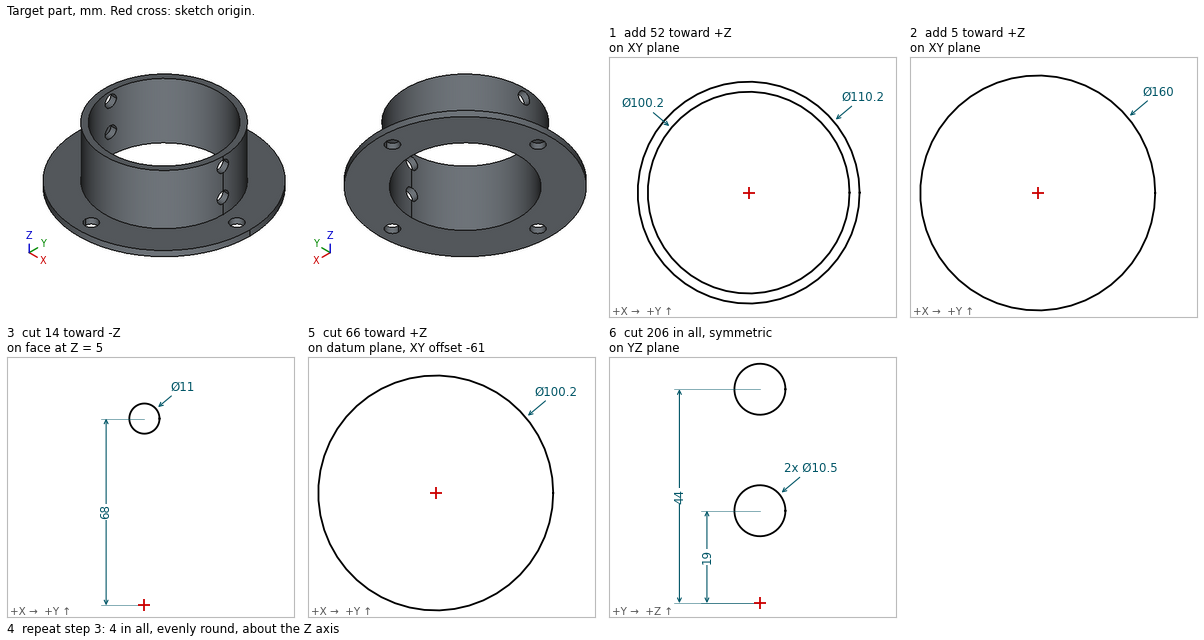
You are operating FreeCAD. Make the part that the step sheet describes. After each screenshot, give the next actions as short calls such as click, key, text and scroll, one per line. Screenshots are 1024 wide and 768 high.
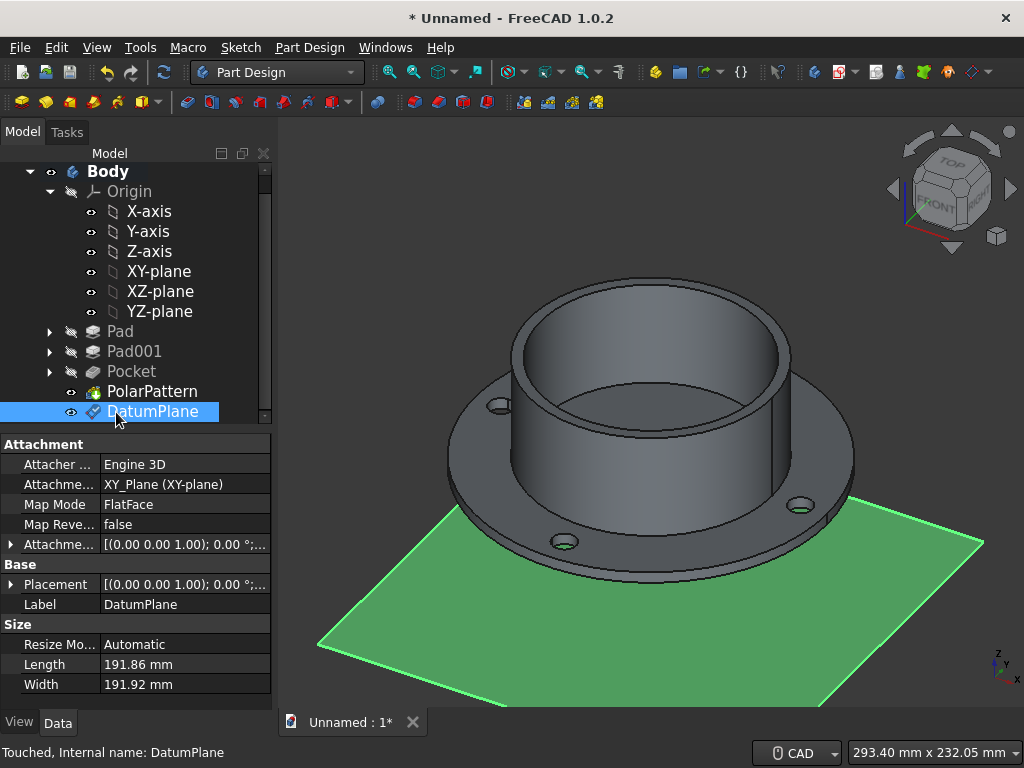
click(840, 72)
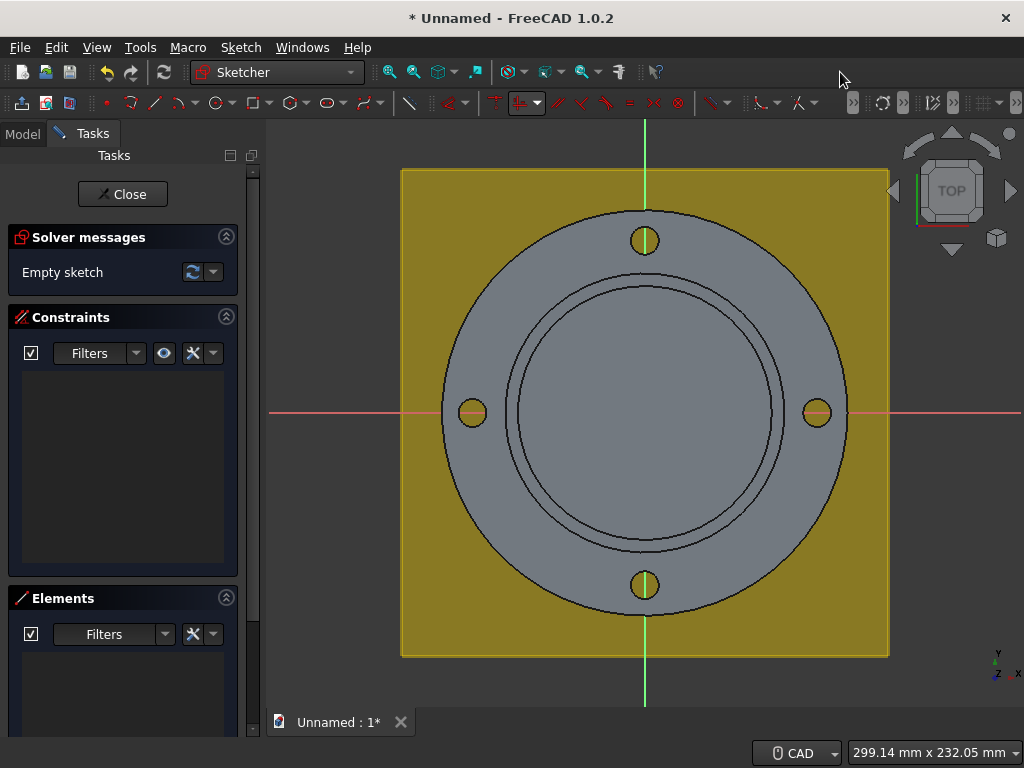
click(70, 104)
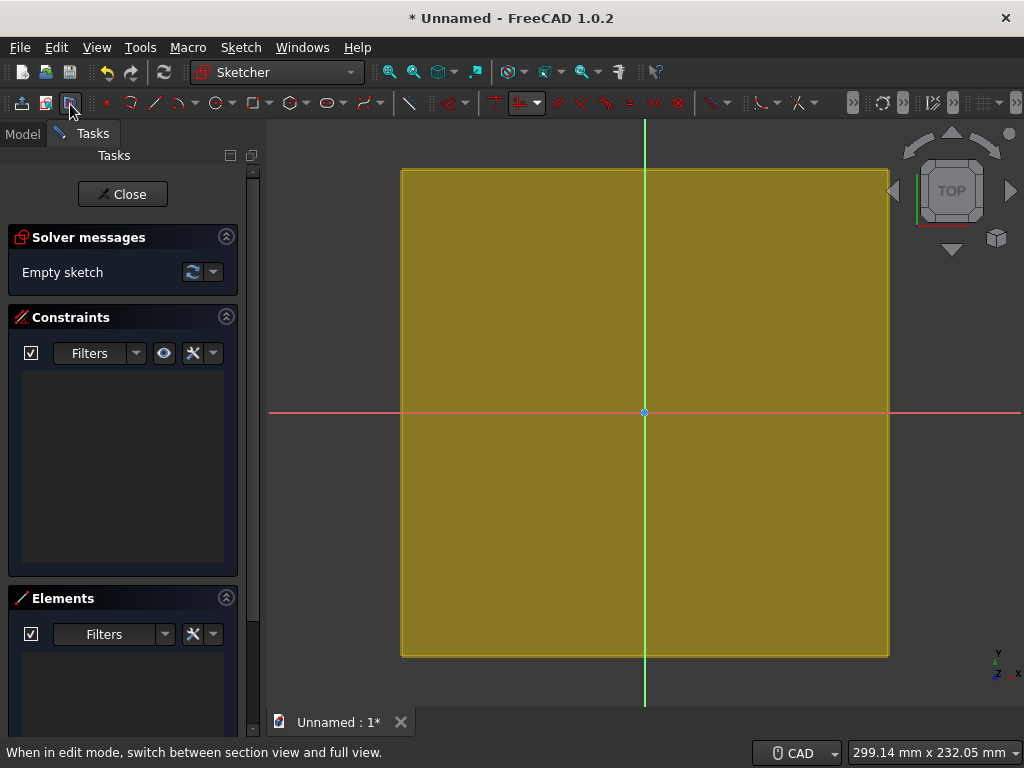
scroll(784, 413, up, 2)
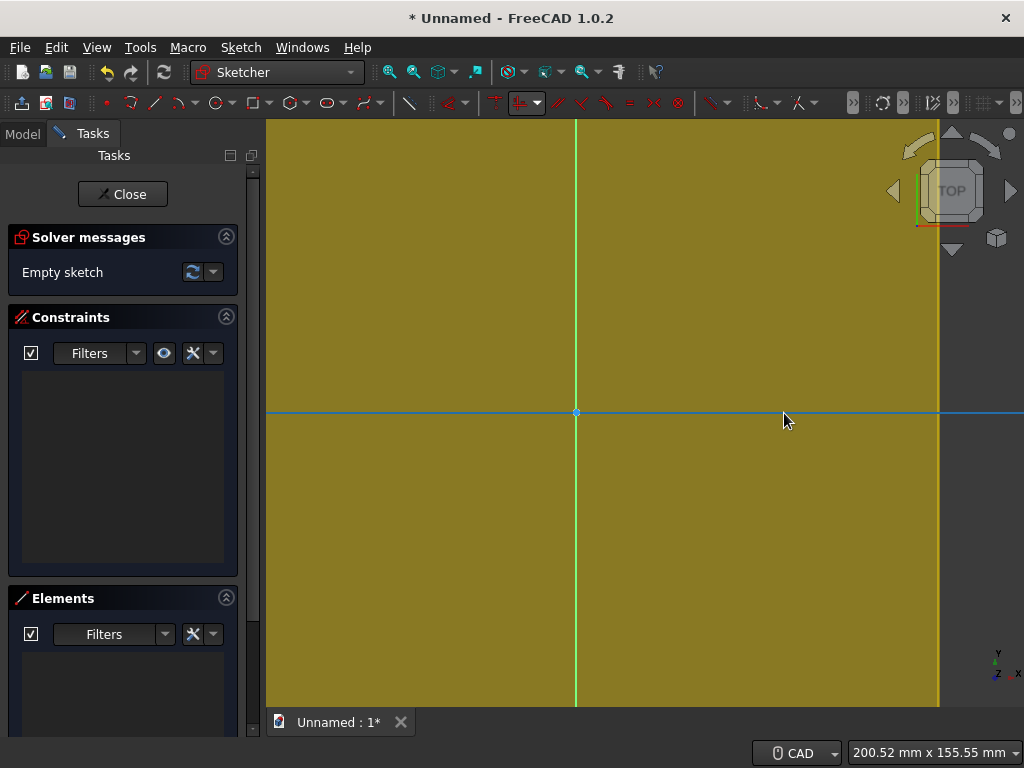
click(216, 104)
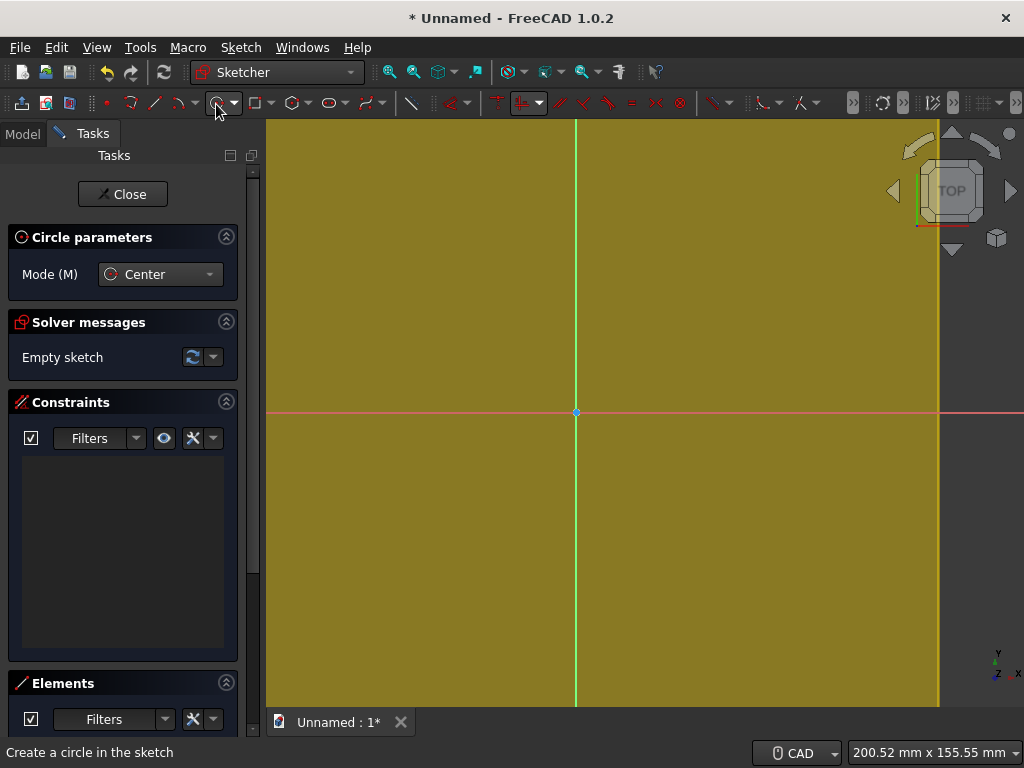
click(576, 413)
click(710, 279)
key(Escape)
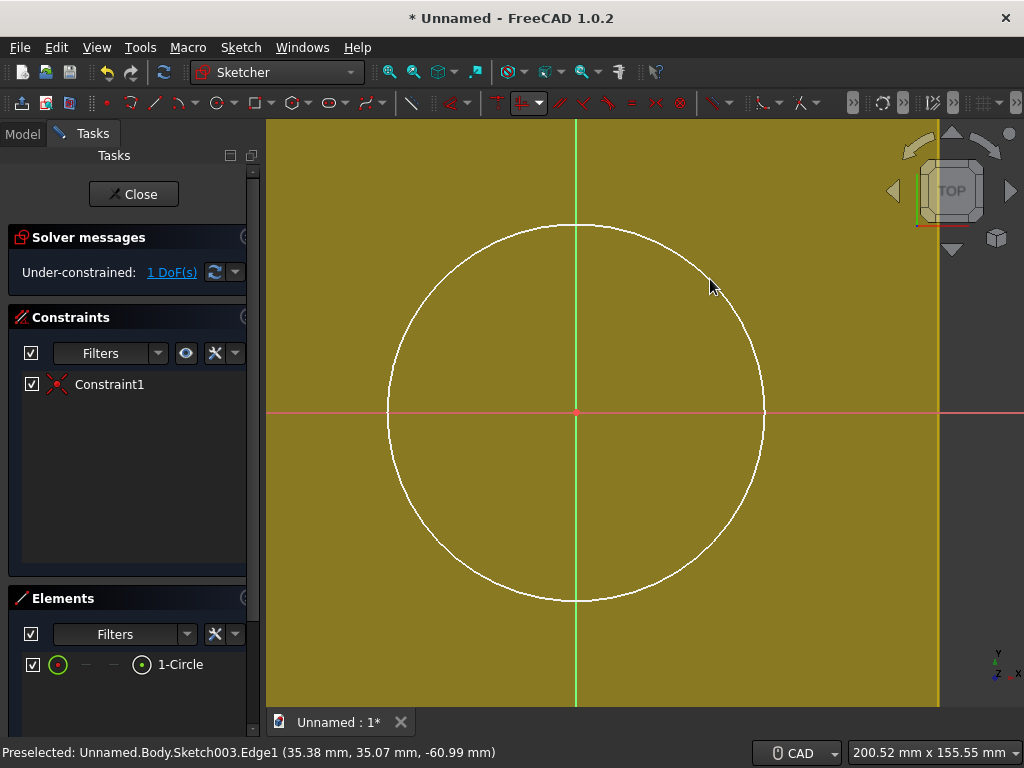
click(450, 104)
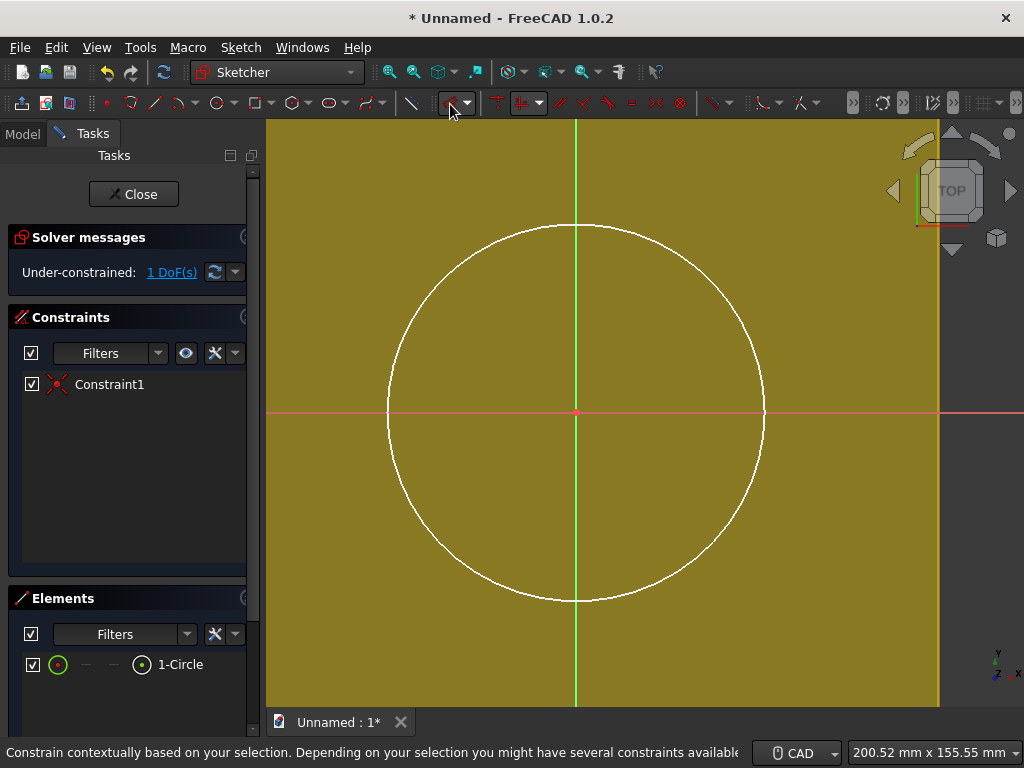
click(709, 279)
click(732, 256)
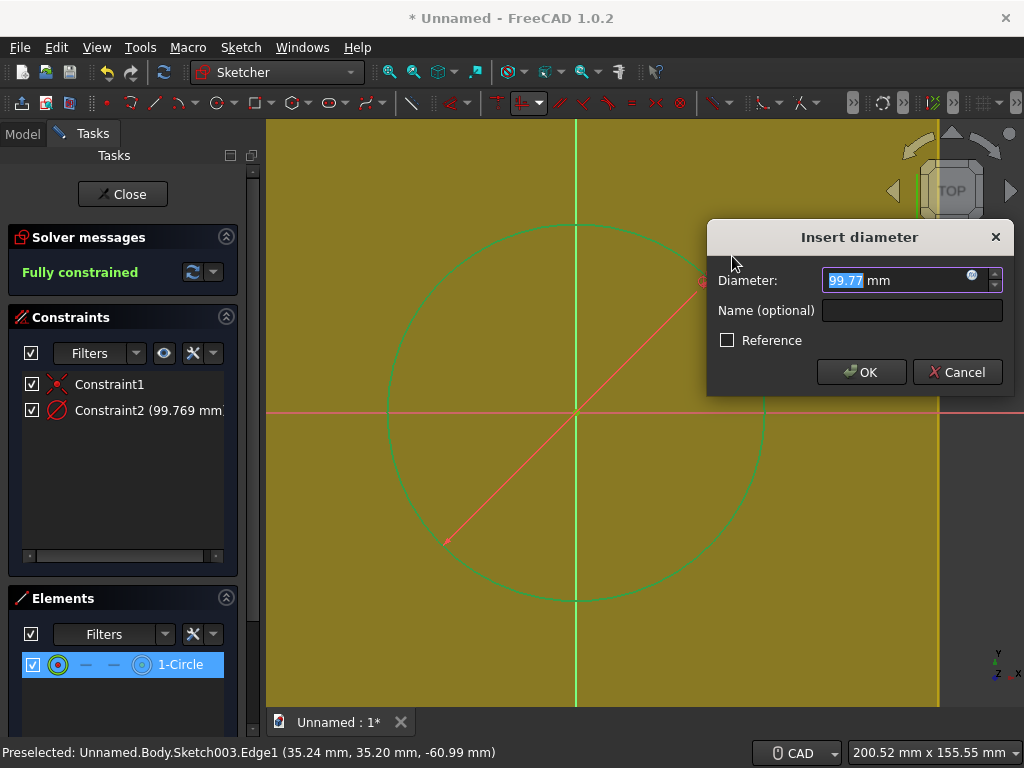
text(100.2)
key(Return)
key(Escape)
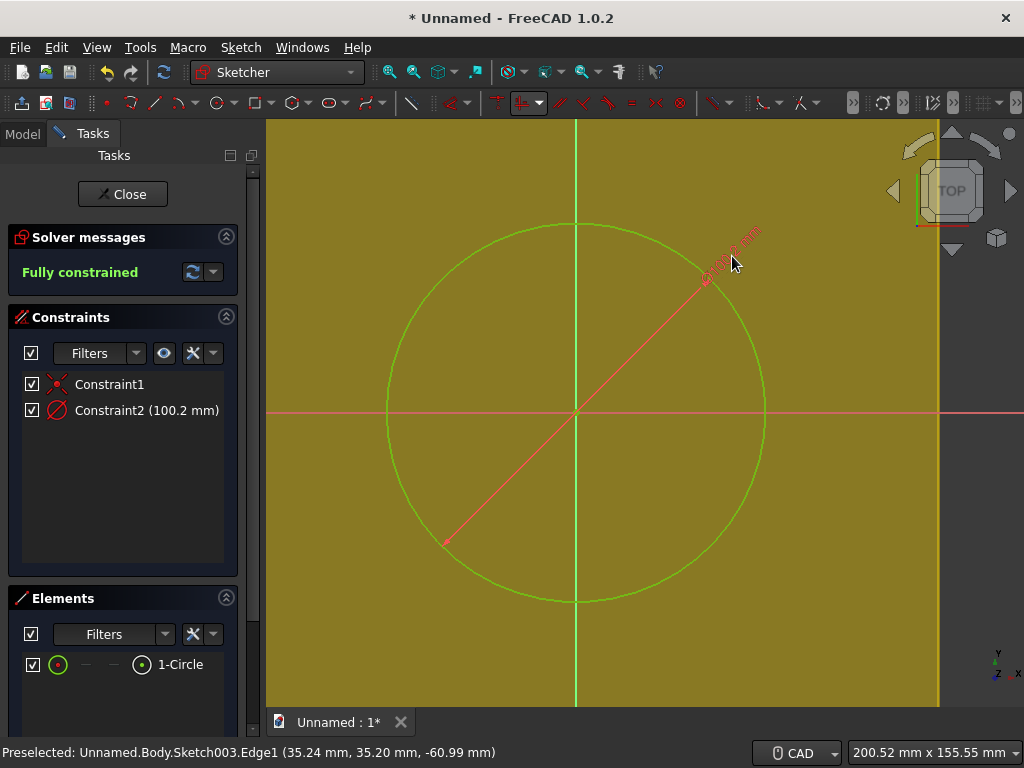
click(123, 194)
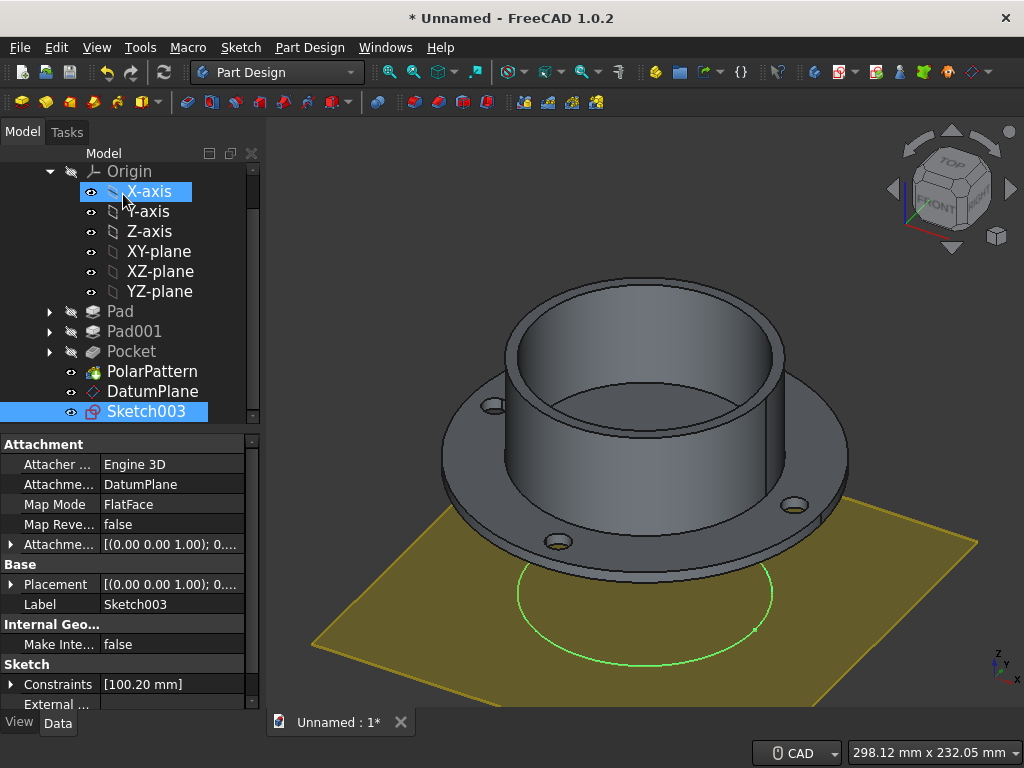
click(188, 102)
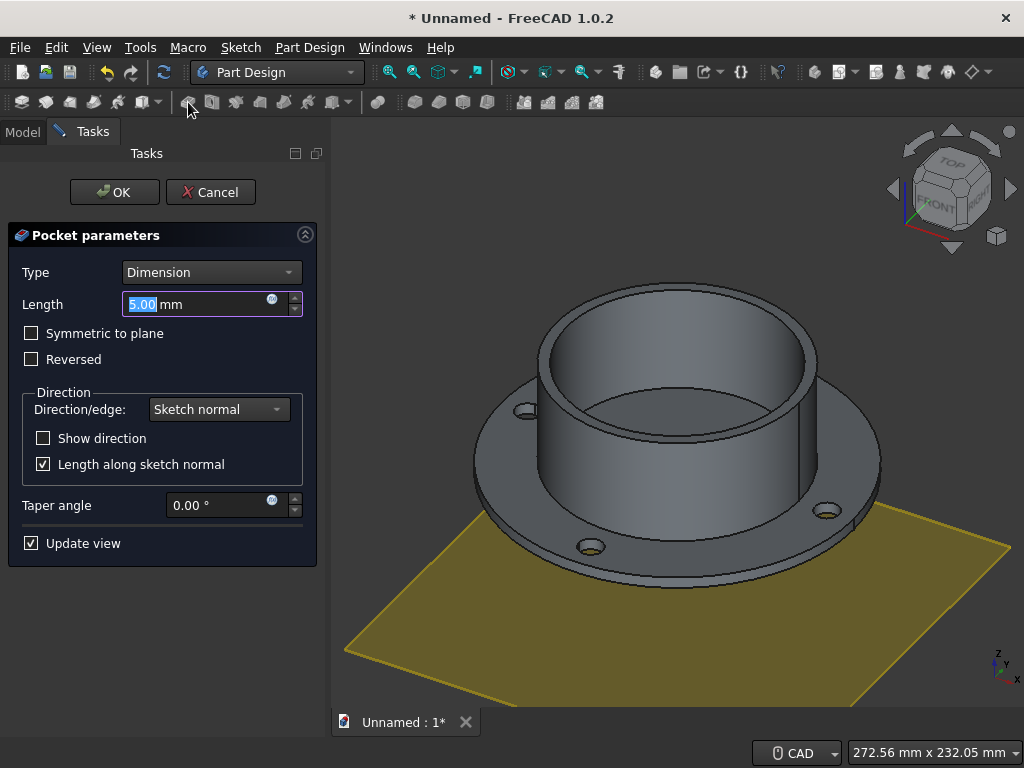
text(66)
key(Tab)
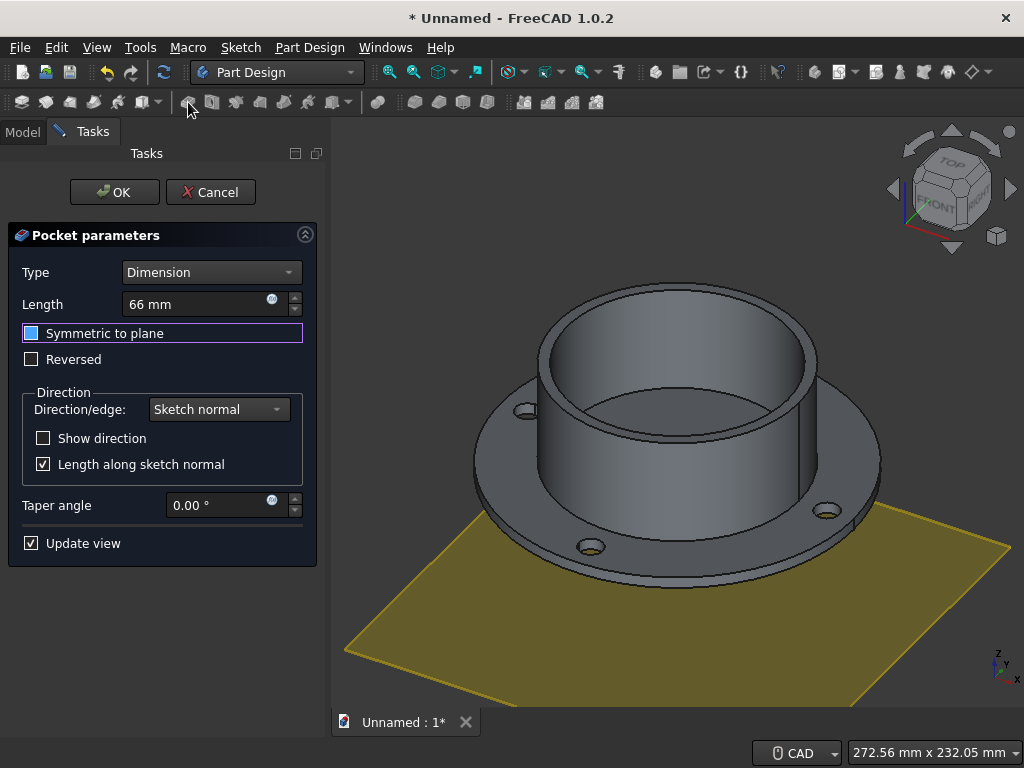
click(30, 359)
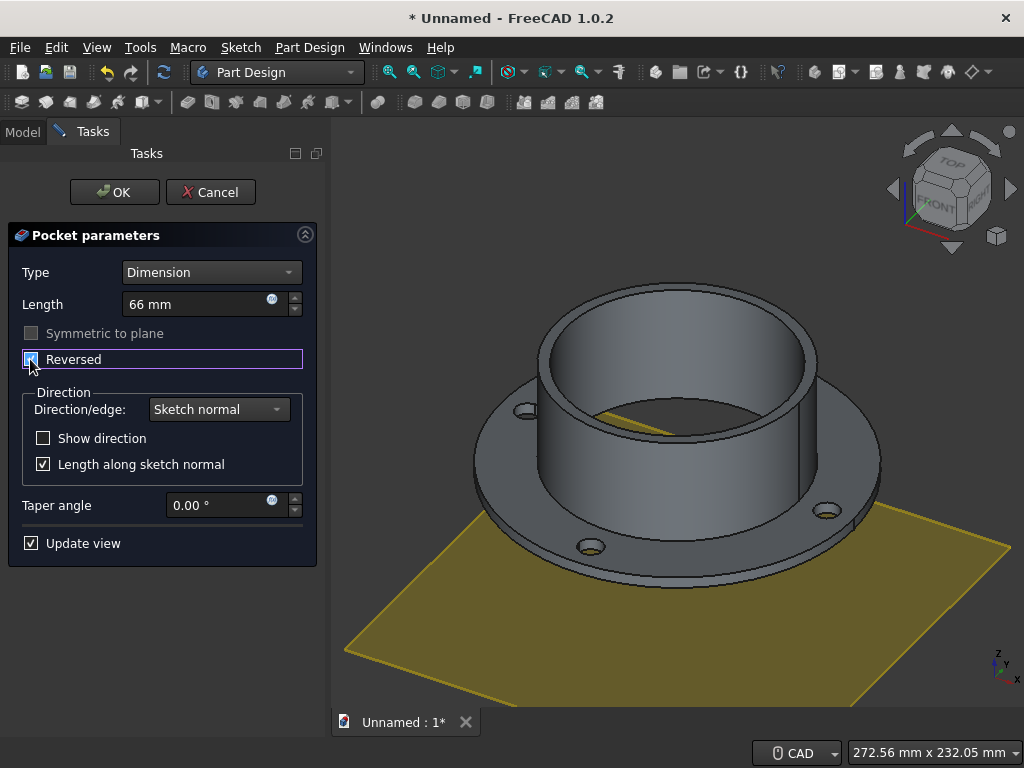
click(115, 192)